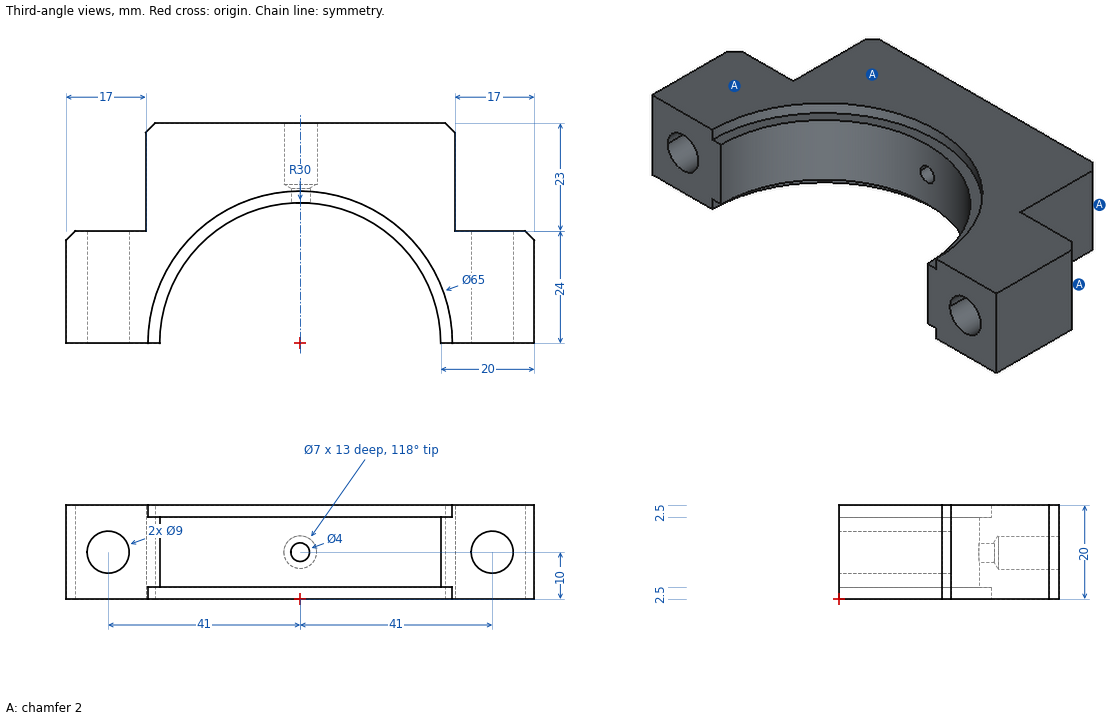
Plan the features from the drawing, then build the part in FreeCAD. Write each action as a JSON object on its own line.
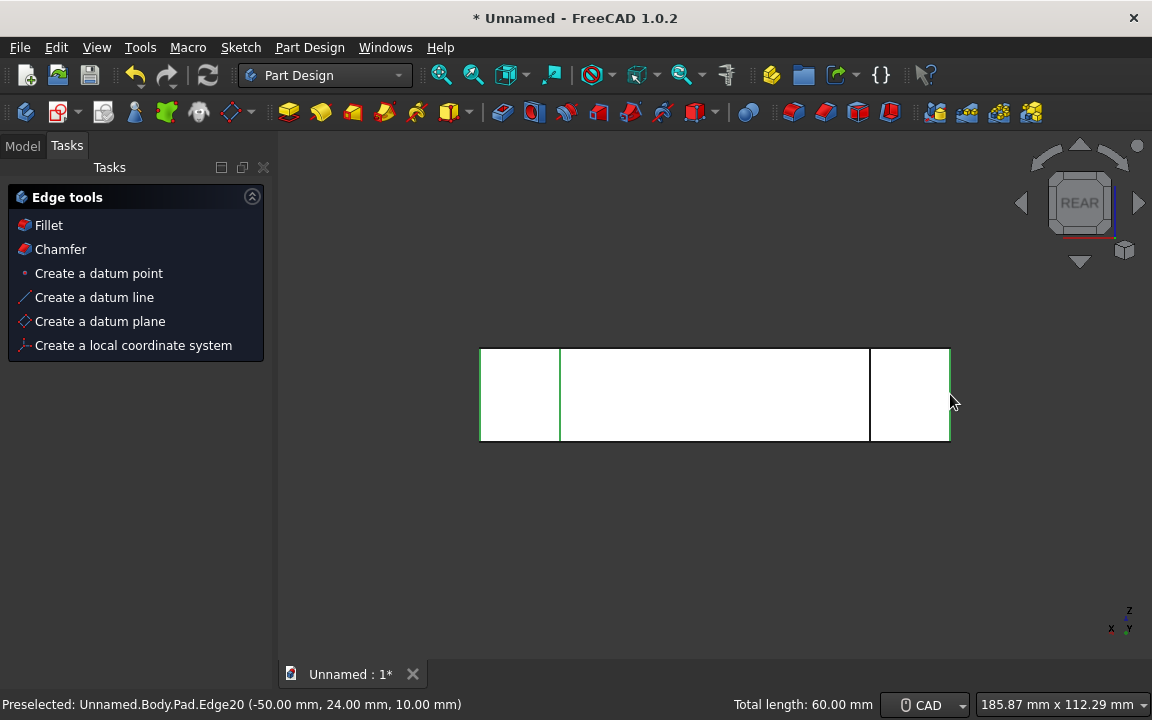
{"action": "left_click", "coordinate": [870, 394], "text": "ctrl"}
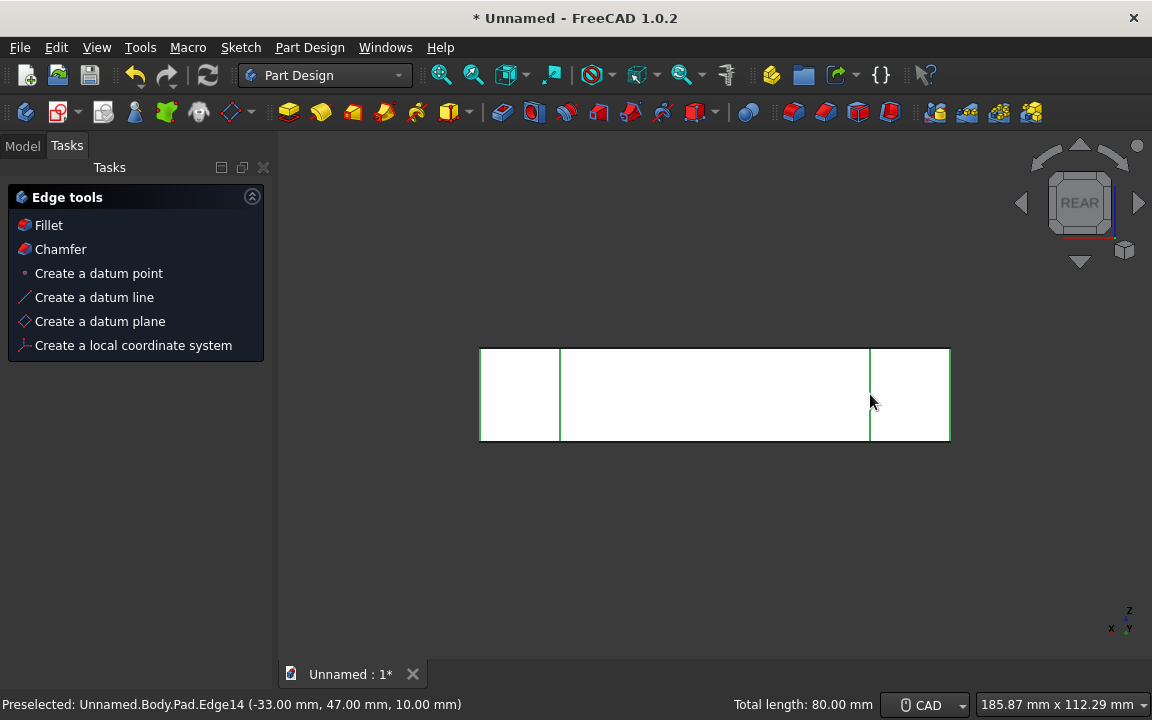
{"action": "left_click", "coordinate": [826, 112]}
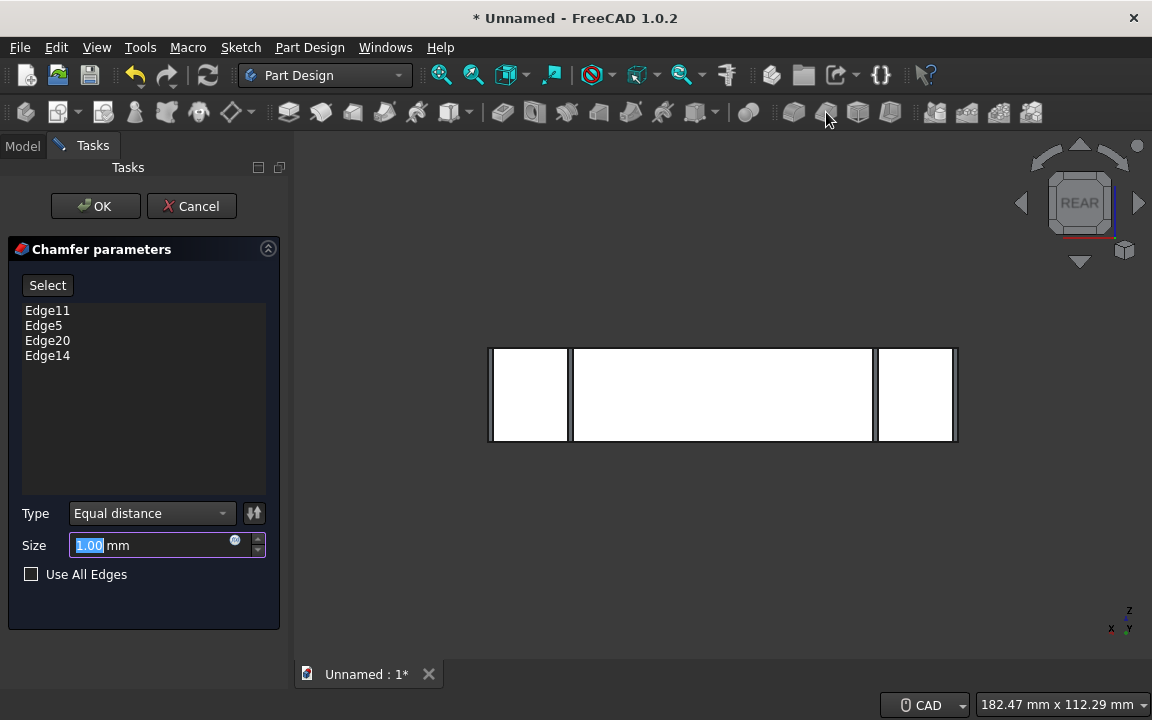
{"action": "type", "text": "2"}
{"action": "key", "text": "Tab"}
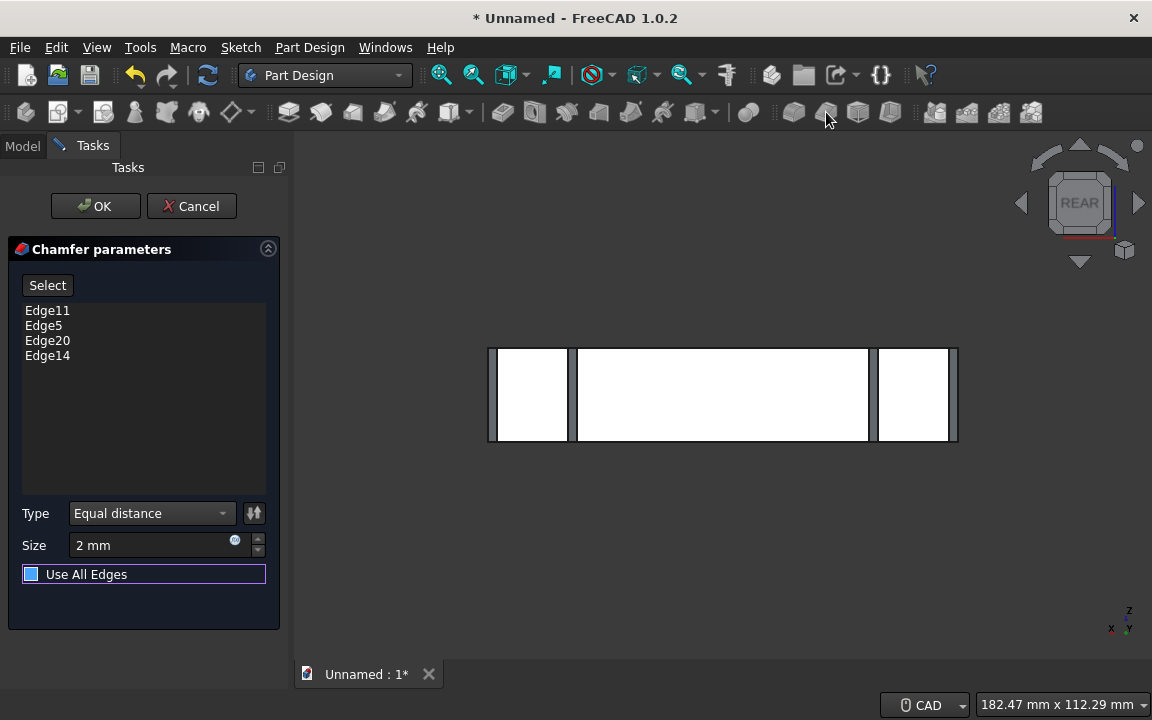
{"action": "left_click", "coordinate": [96, 206]}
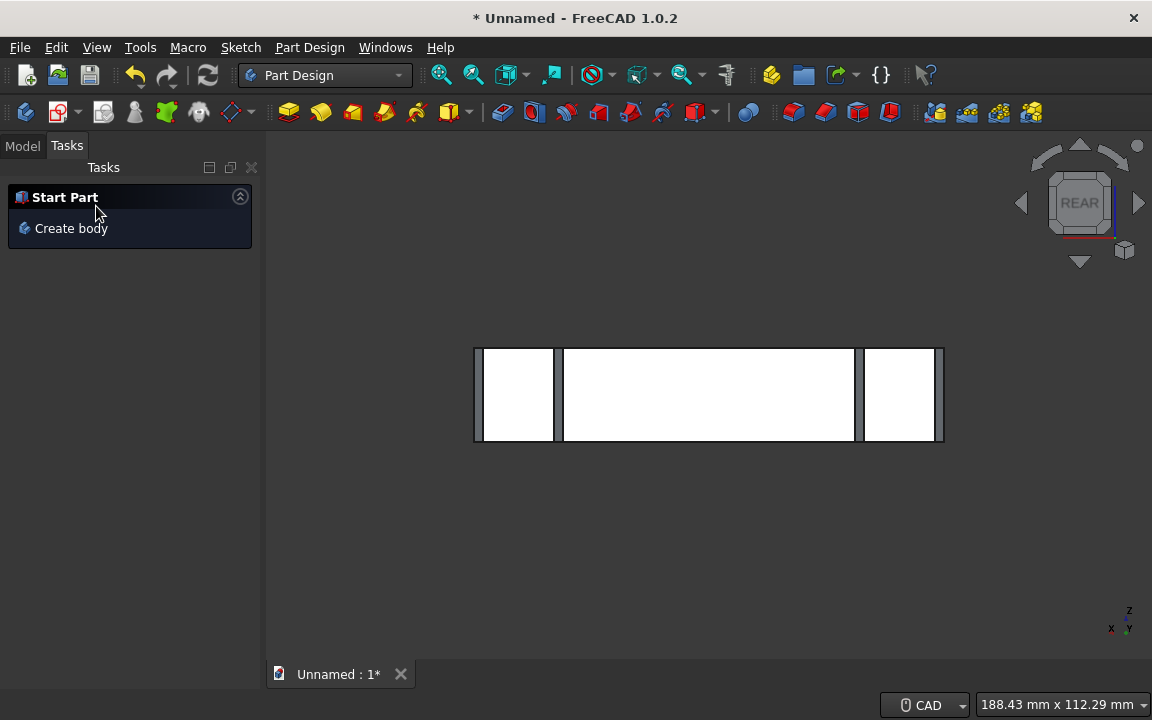
{"action": "left_click", "coordinate": [626, 394]}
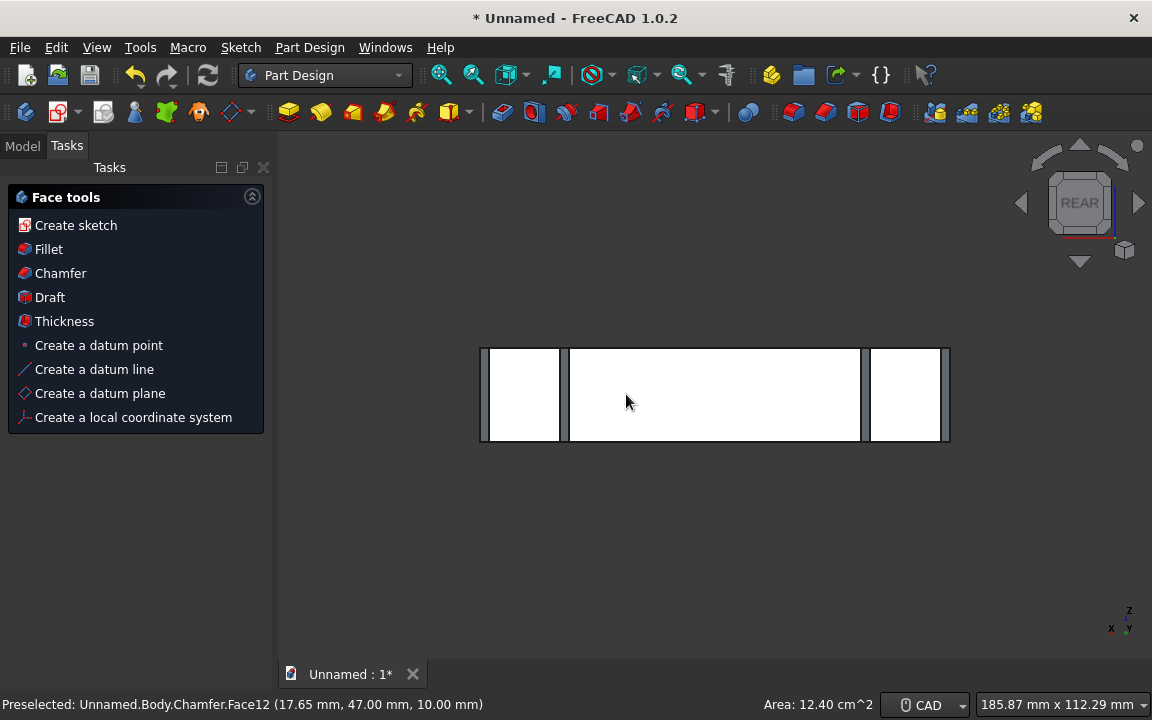
{"action": "left_click", "coordinate": [58, 112]}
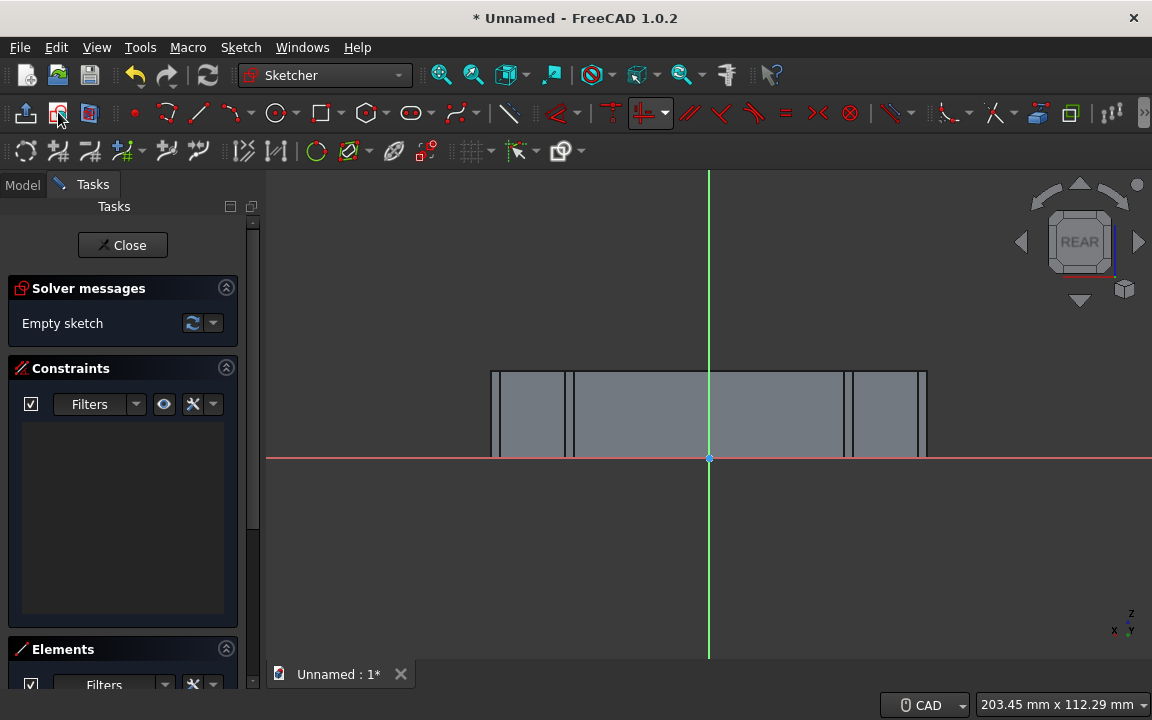
{"action": "scroll", "coordinate": [726, 432], "scroll_direction": "up", "scroll_amount": 8}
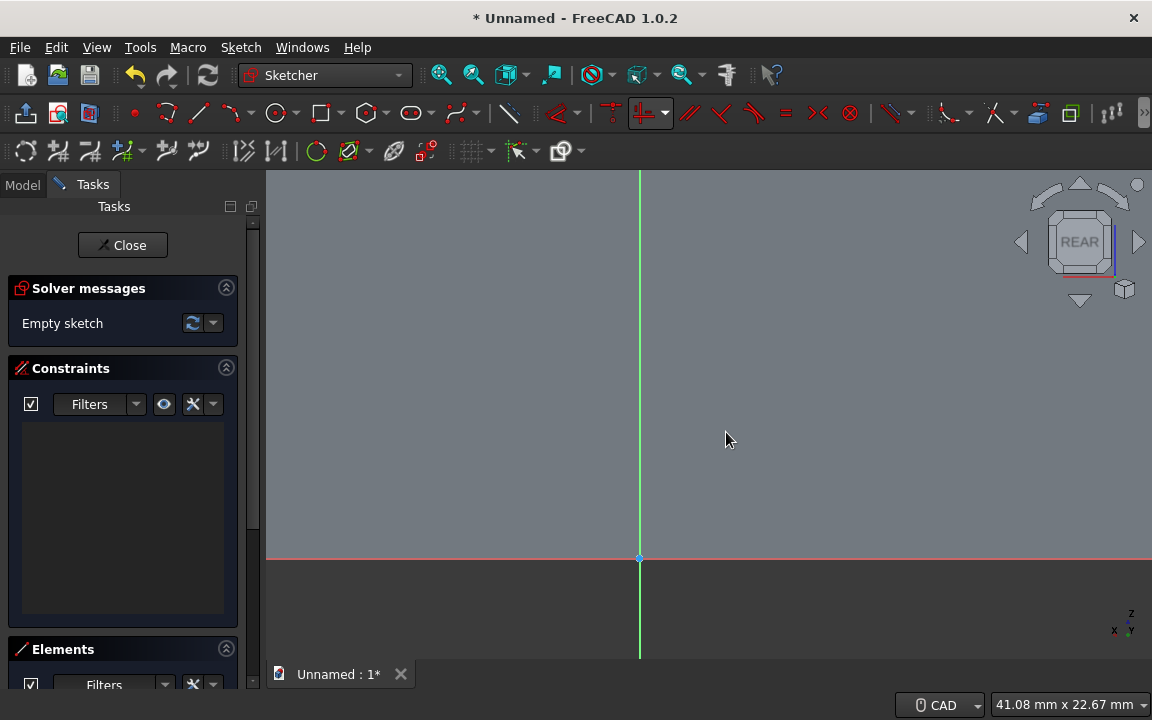
{"action": "left_click", "coordinate": [276, 114]}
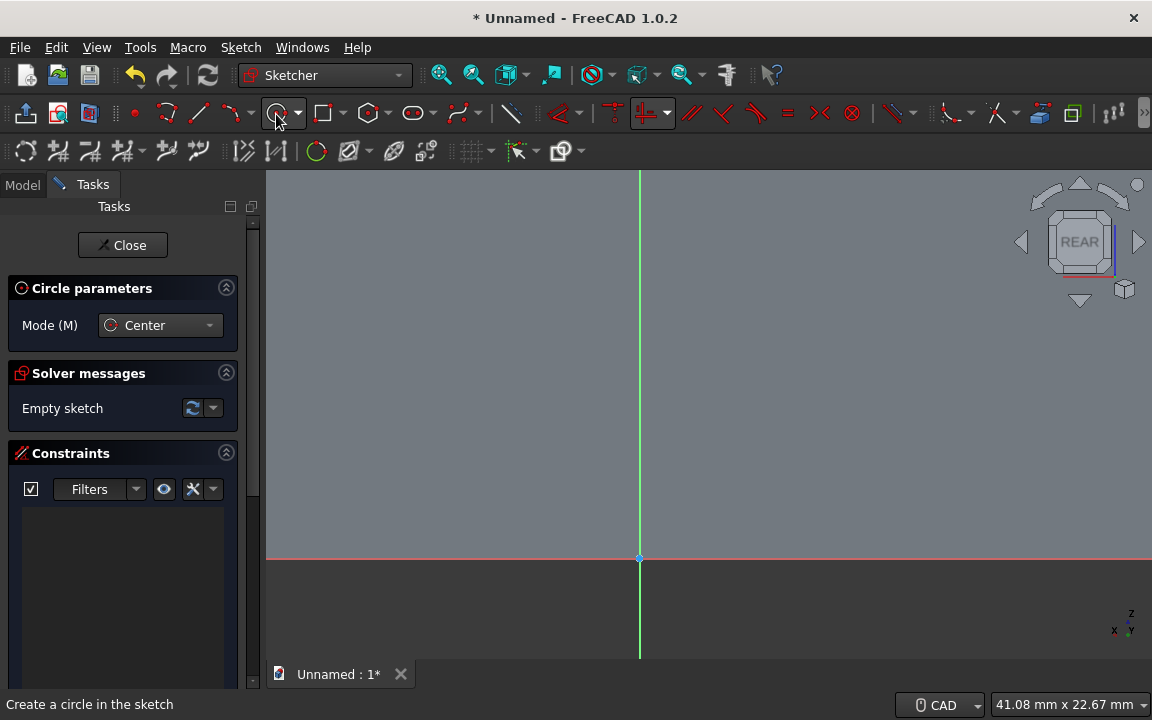
{"action": "left_click", "coordinate": [640, 343]}
{"action": "mouse_move", "coordinate": [693, 290]}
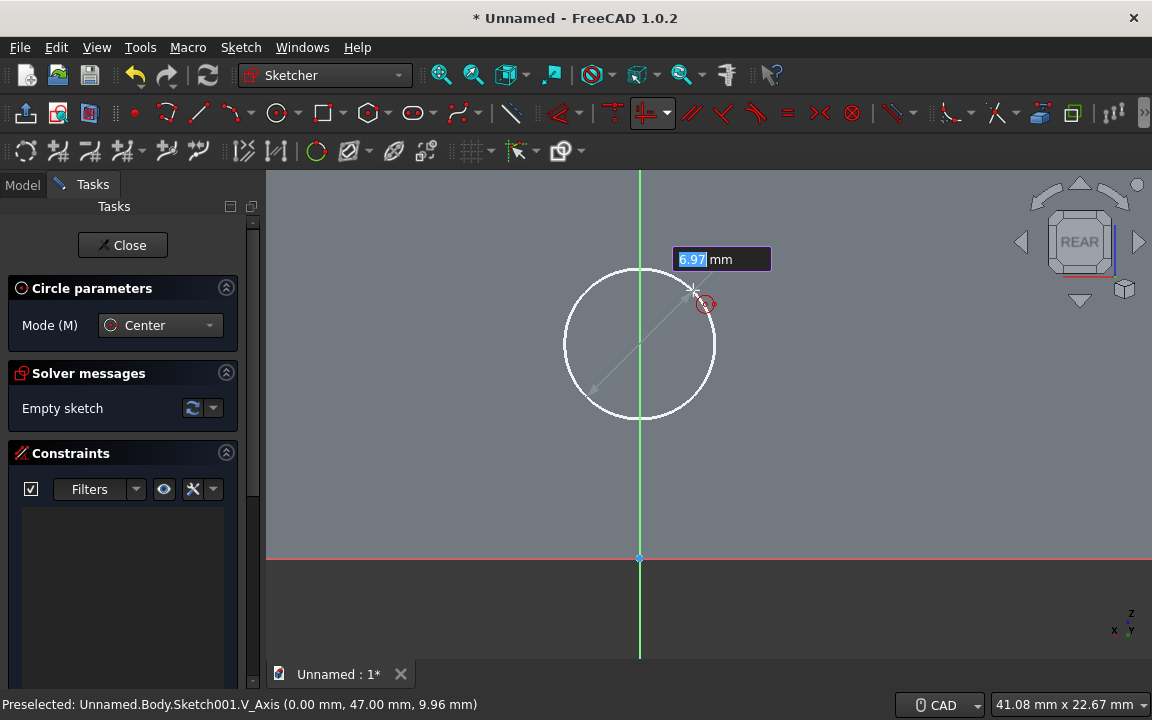
{"action": "type", "text": "7"}
{"action": "key", "text": "Return"}
{"action": "key", "text": "Escape"}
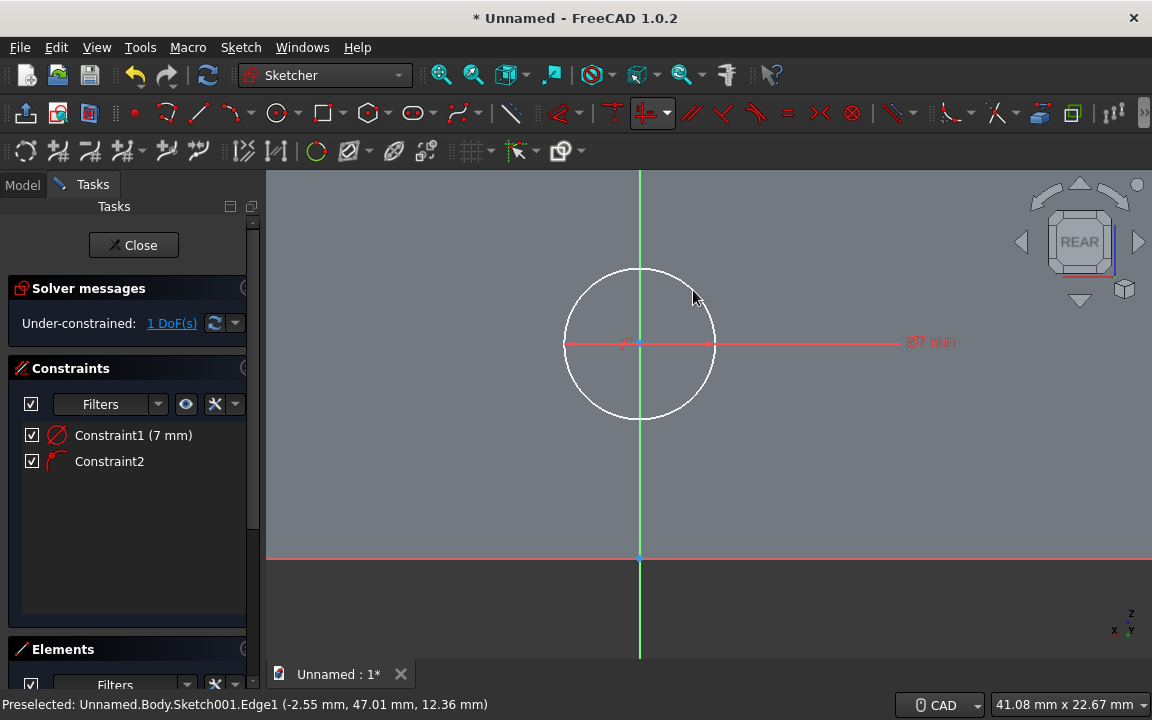
{"action": "left_click", "coordinate": [558, 114]}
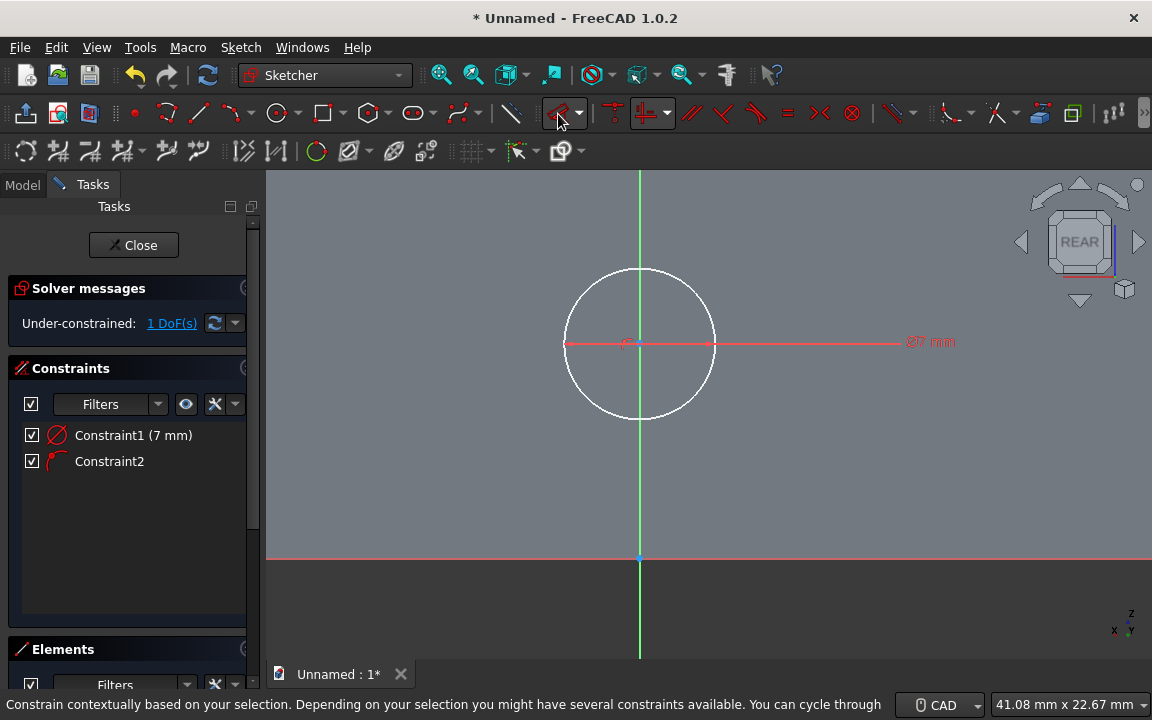
{"action": "left_click", "coordinate": [640, 344]}
{"action": "left_click", "coordinate": [674, 451]}